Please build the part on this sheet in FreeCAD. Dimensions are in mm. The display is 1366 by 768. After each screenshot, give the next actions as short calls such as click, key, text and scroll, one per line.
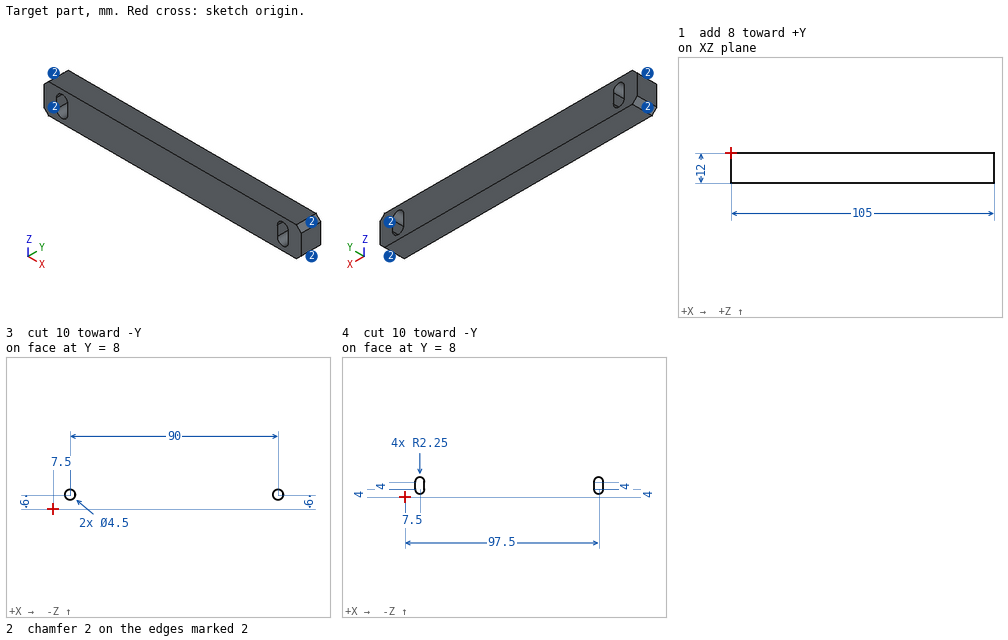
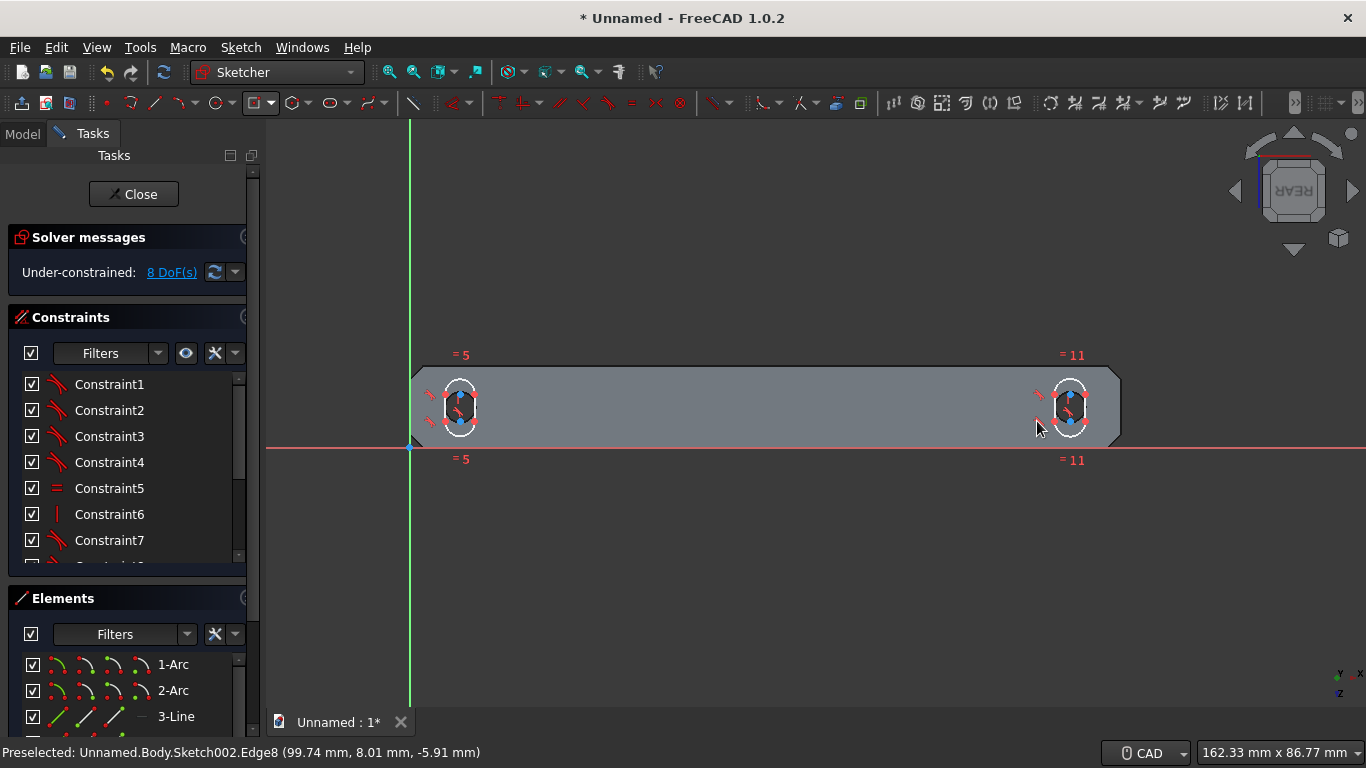
click(451, 433)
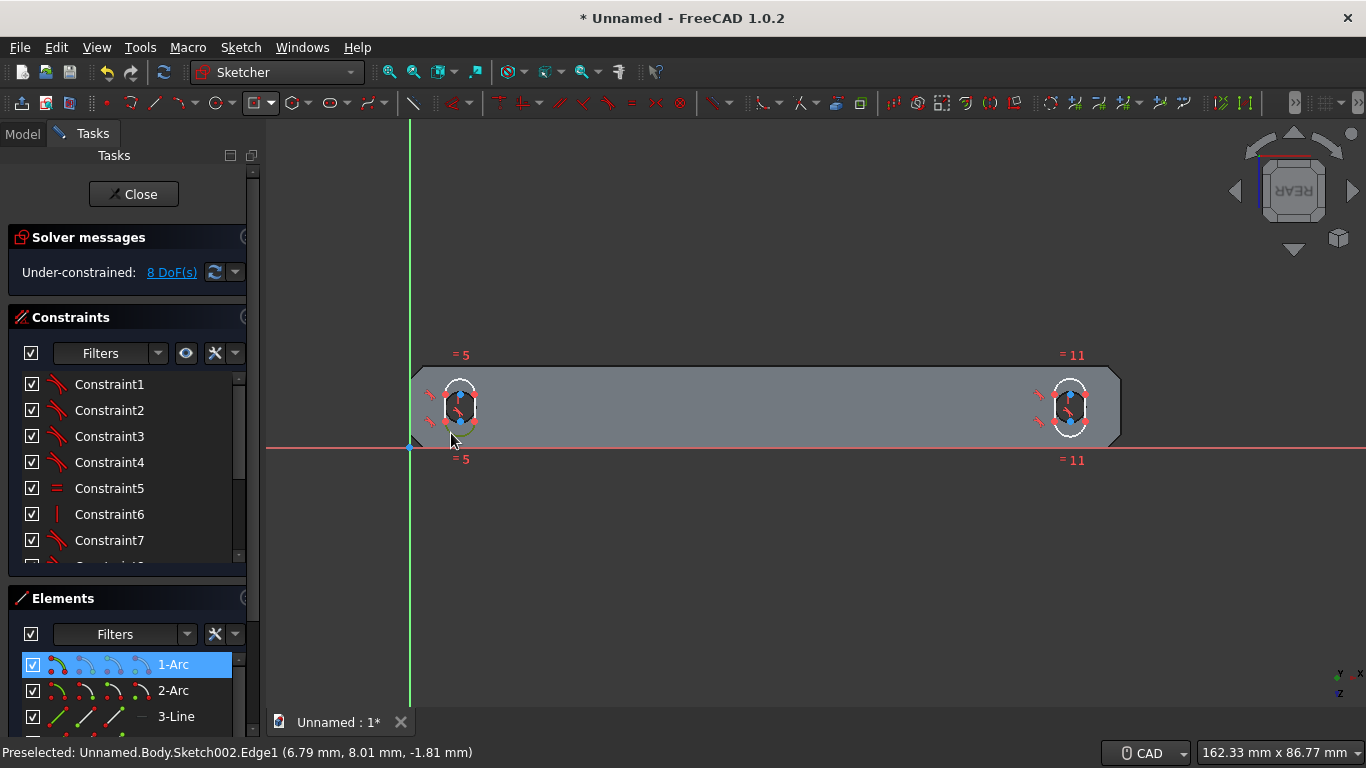
click(1061, 434)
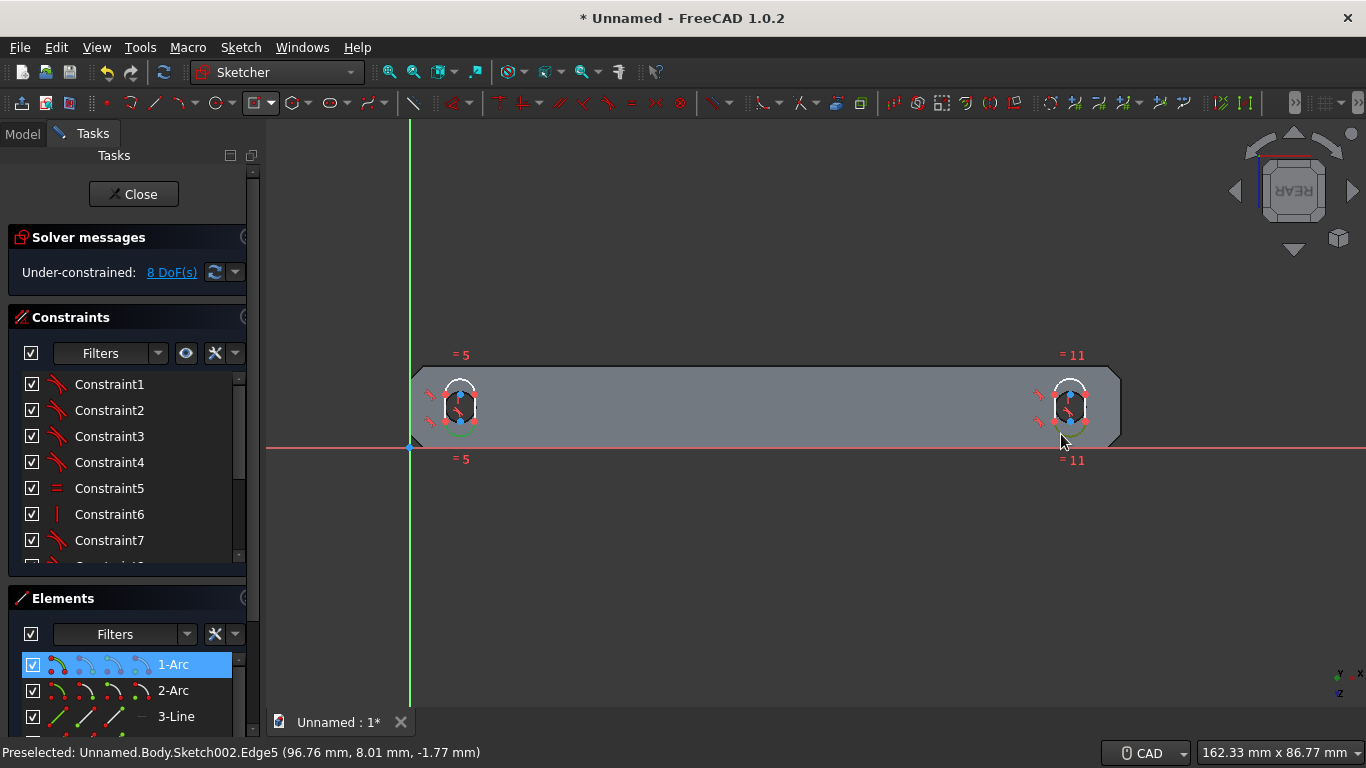
click(632, 104)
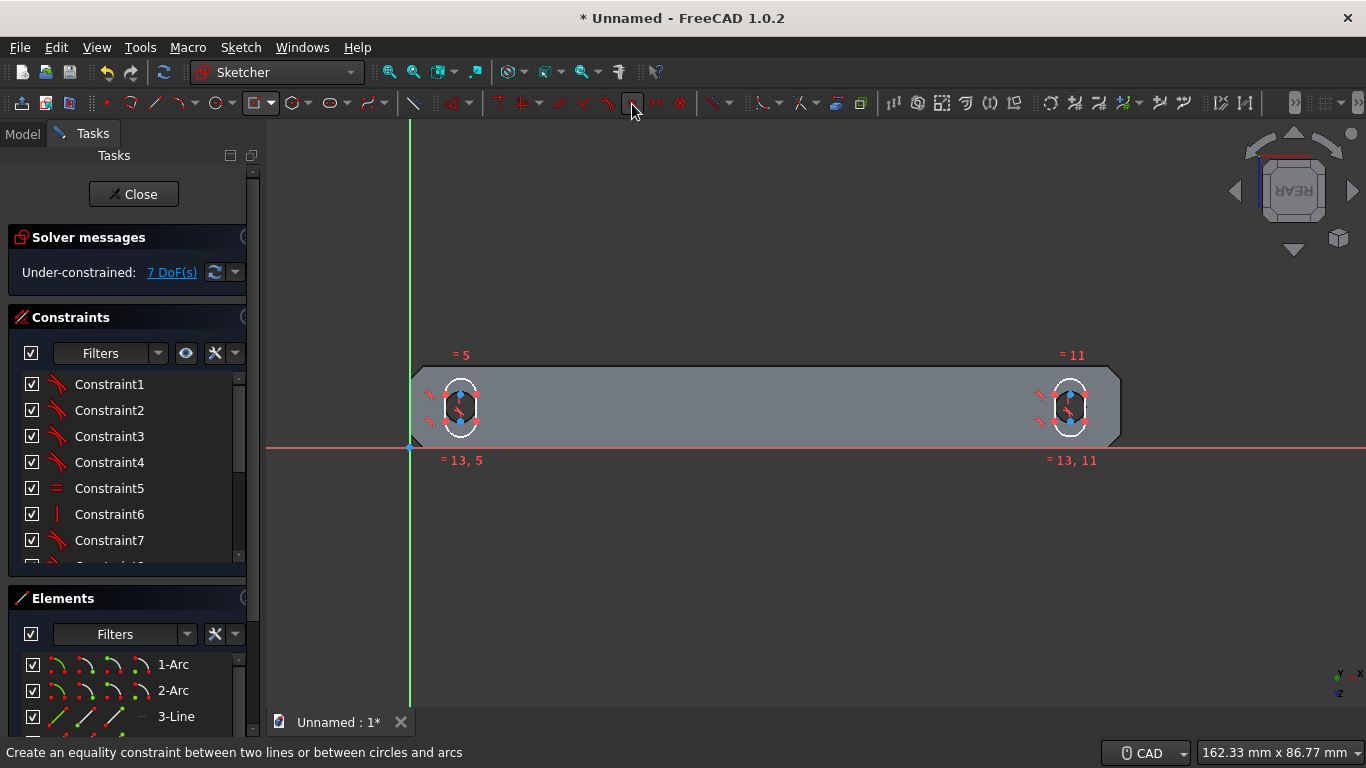
click(452, 104)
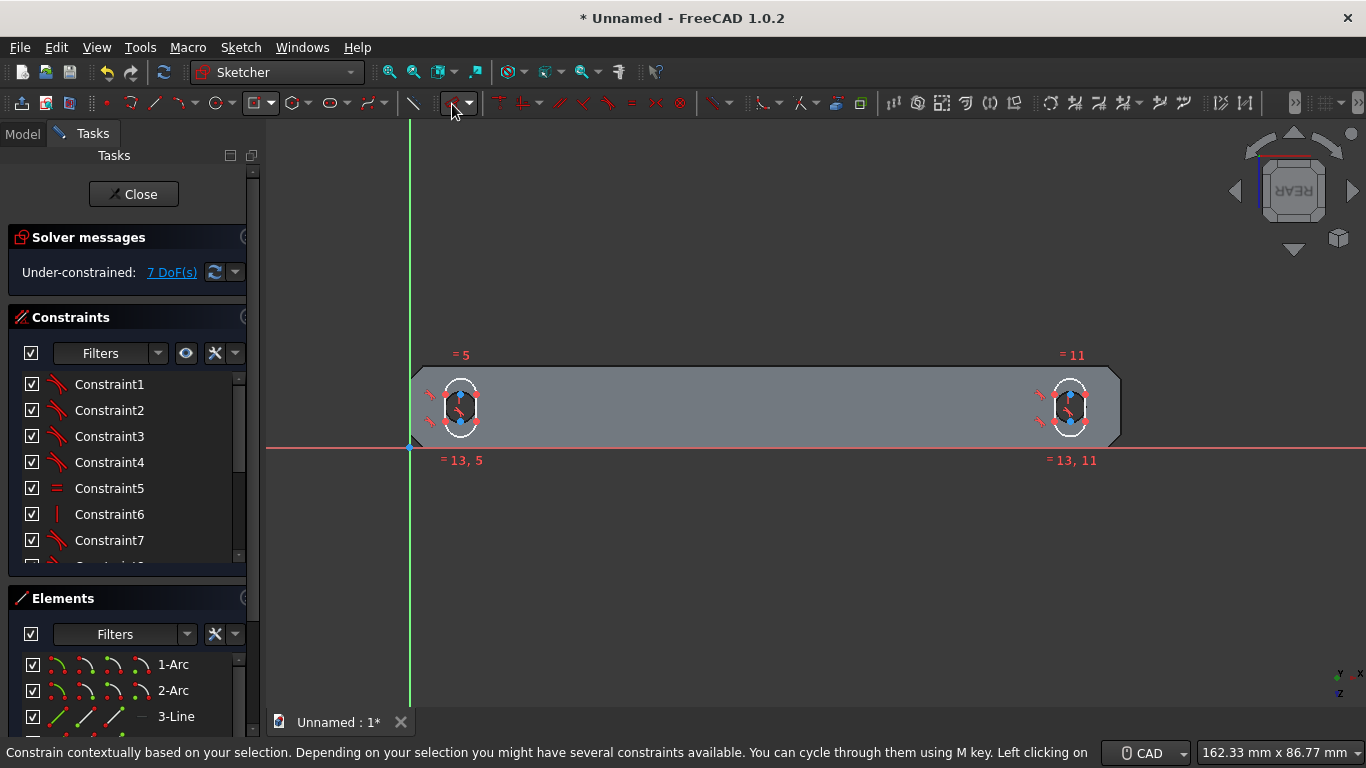
scroll(452, 434, up, 5)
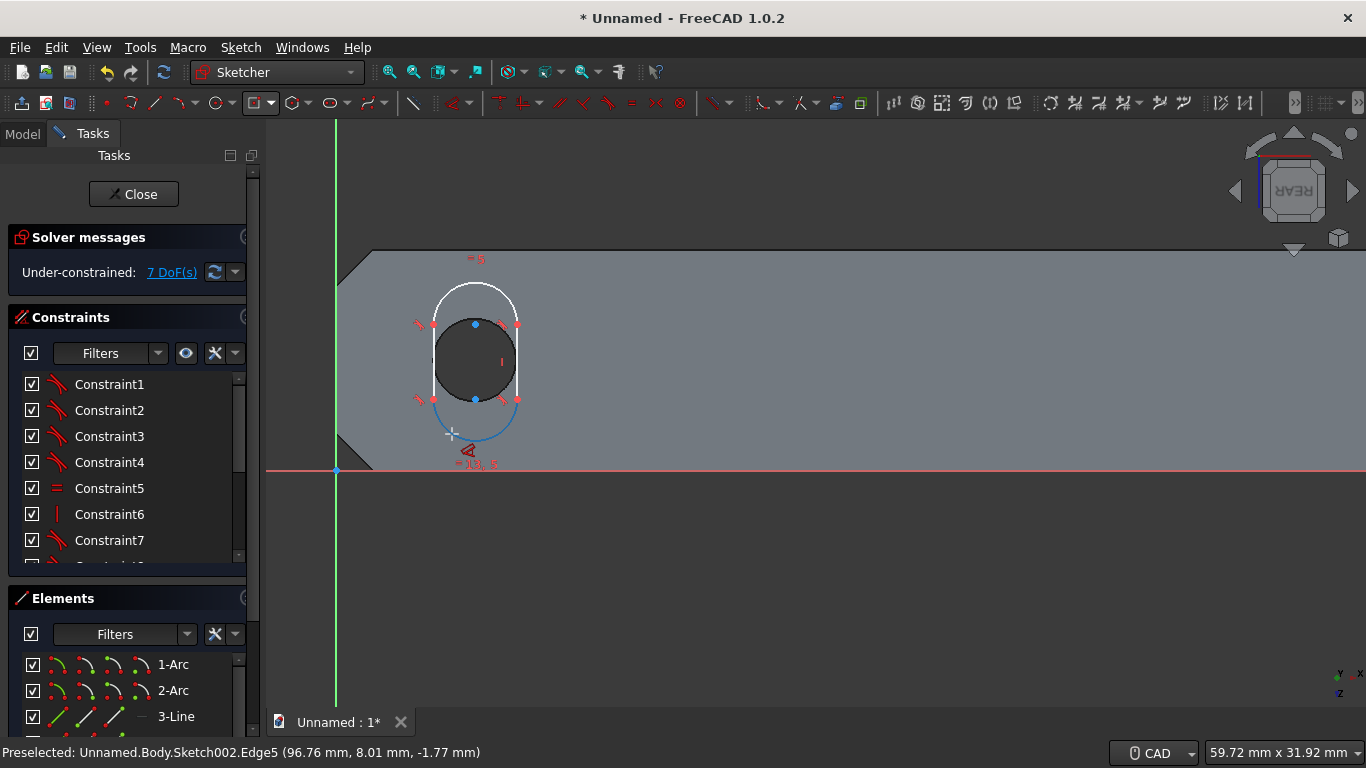
click(451, 433)
click(409, 431)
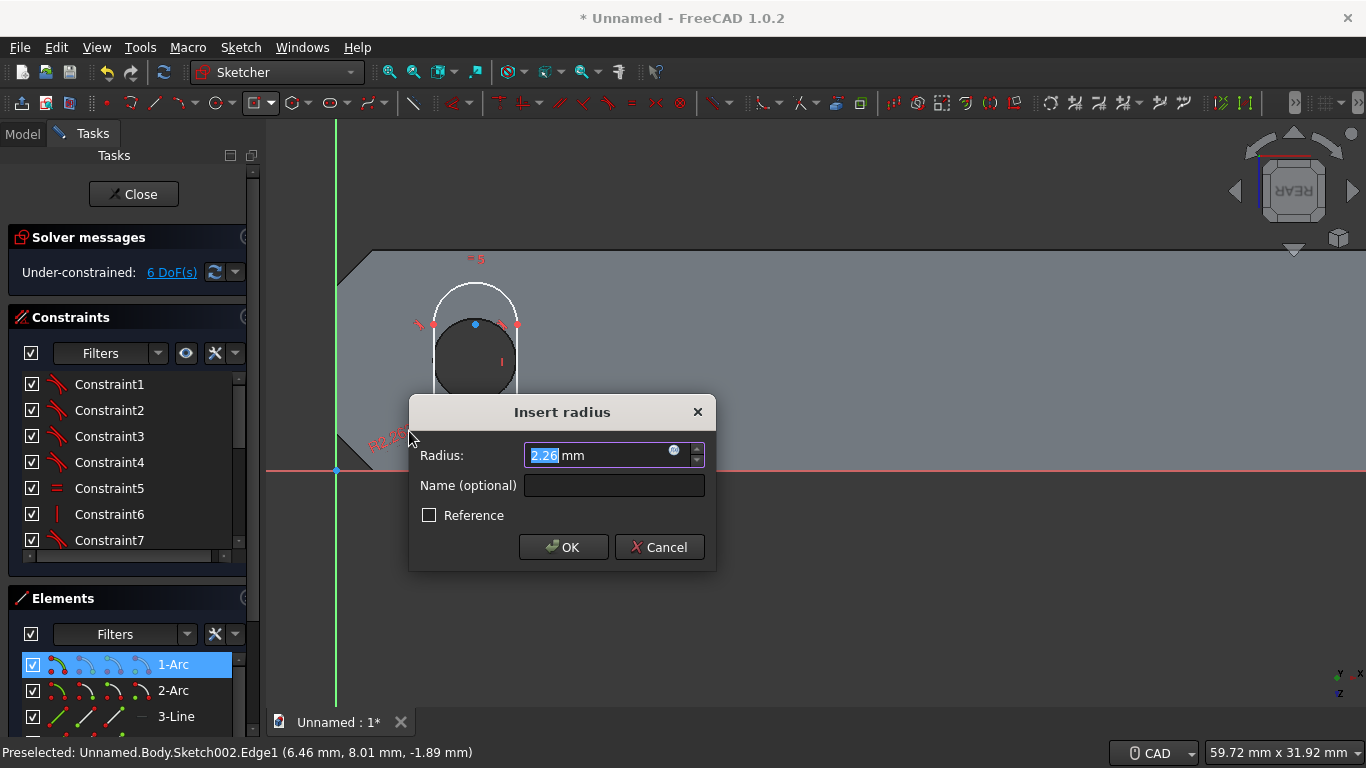
text(2.25)
key(Return)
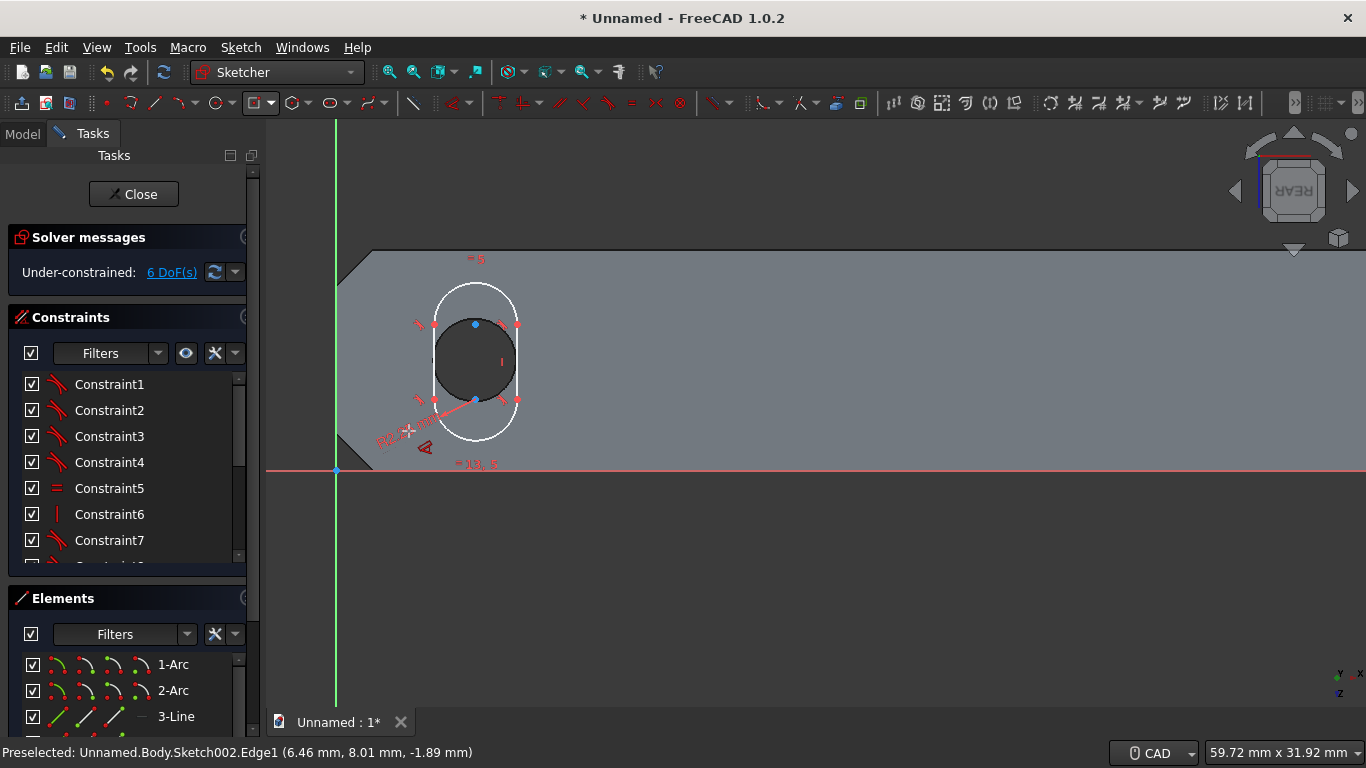
click(434, 377)
click(400, 362)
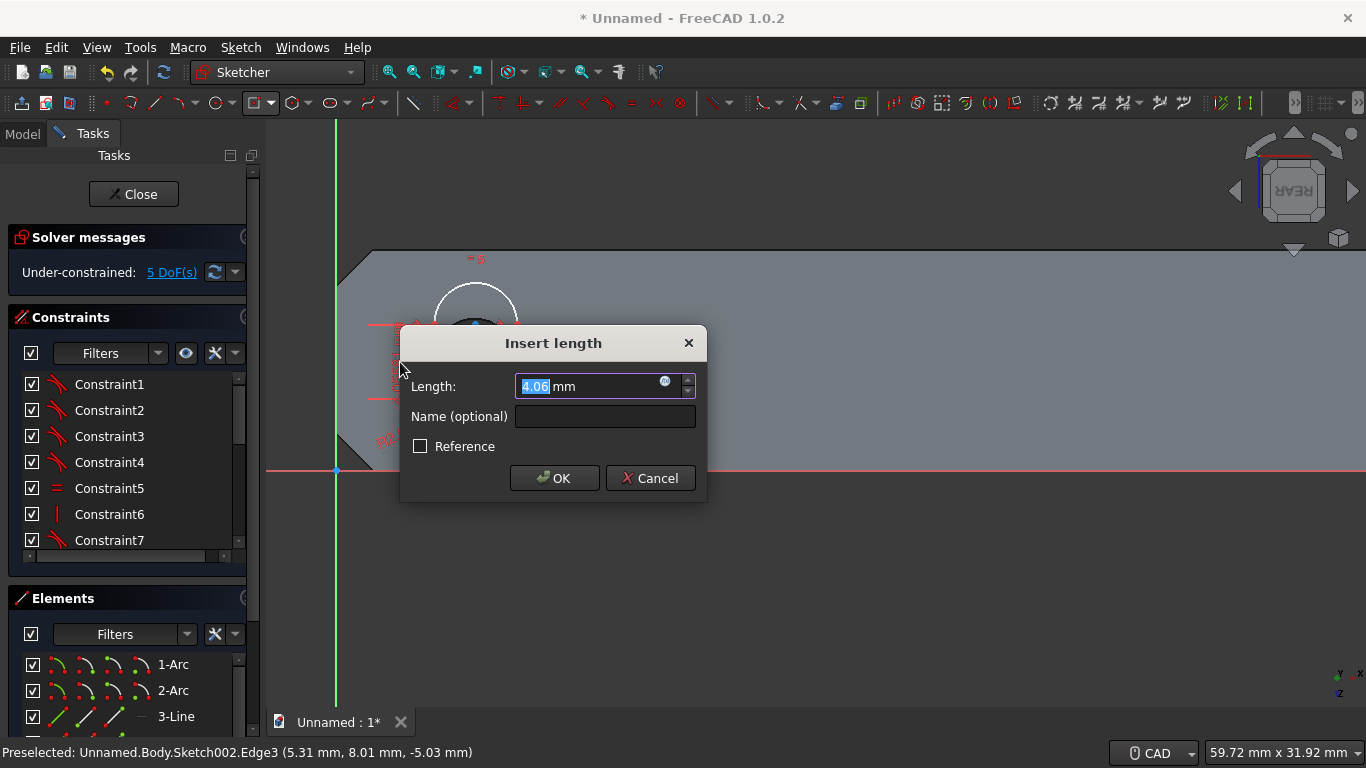
text(4)
key(Return)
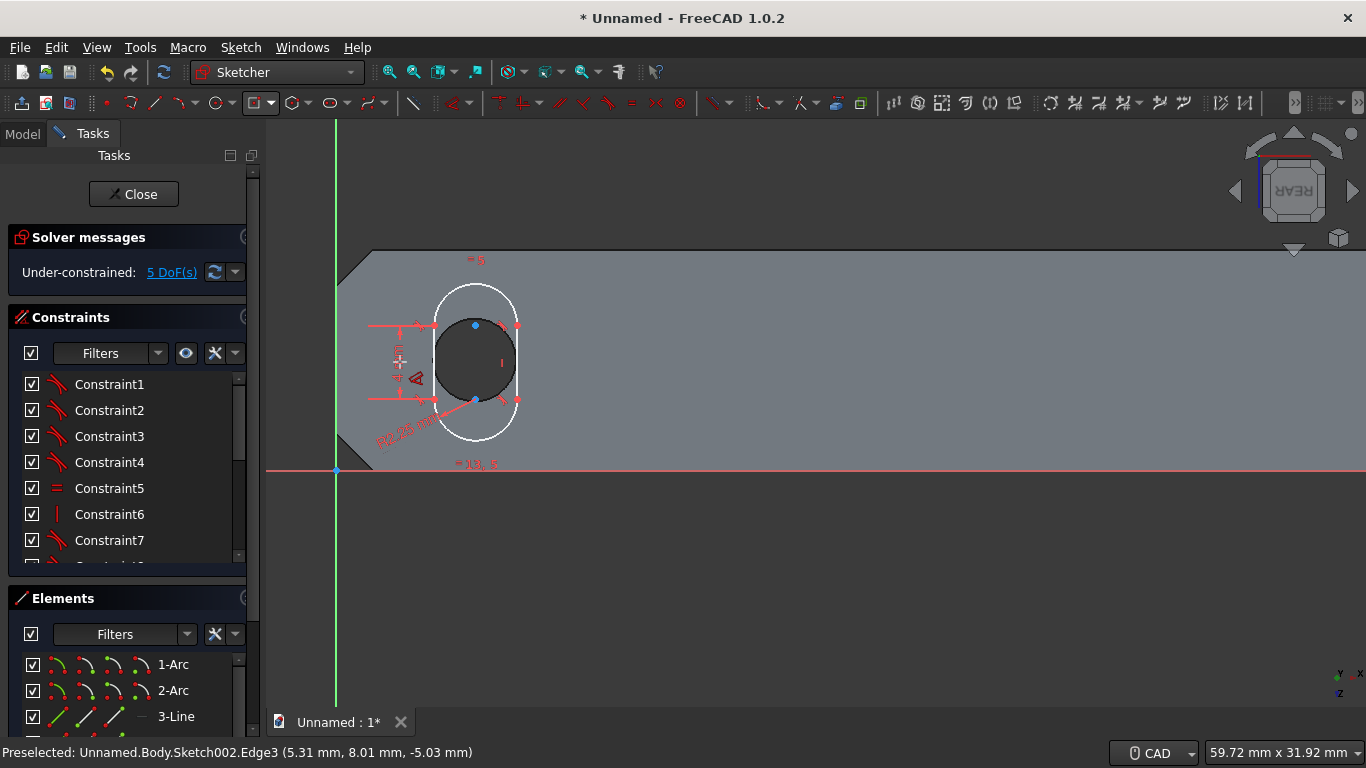
scroll(452, 434, down, 5)